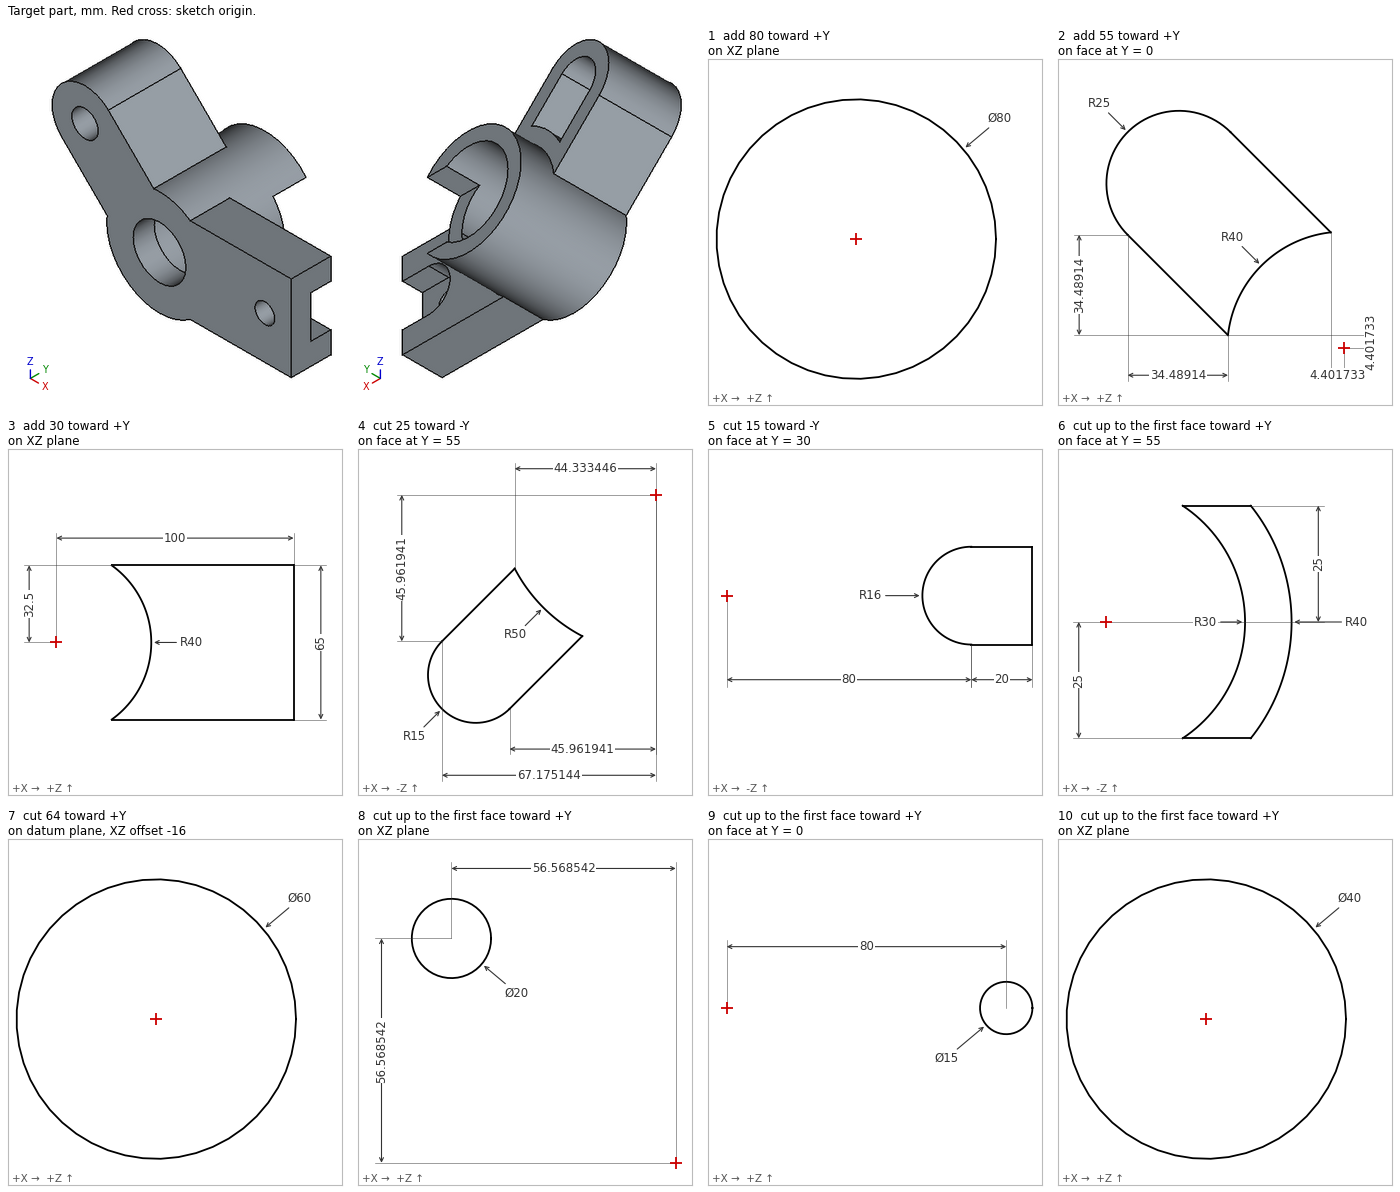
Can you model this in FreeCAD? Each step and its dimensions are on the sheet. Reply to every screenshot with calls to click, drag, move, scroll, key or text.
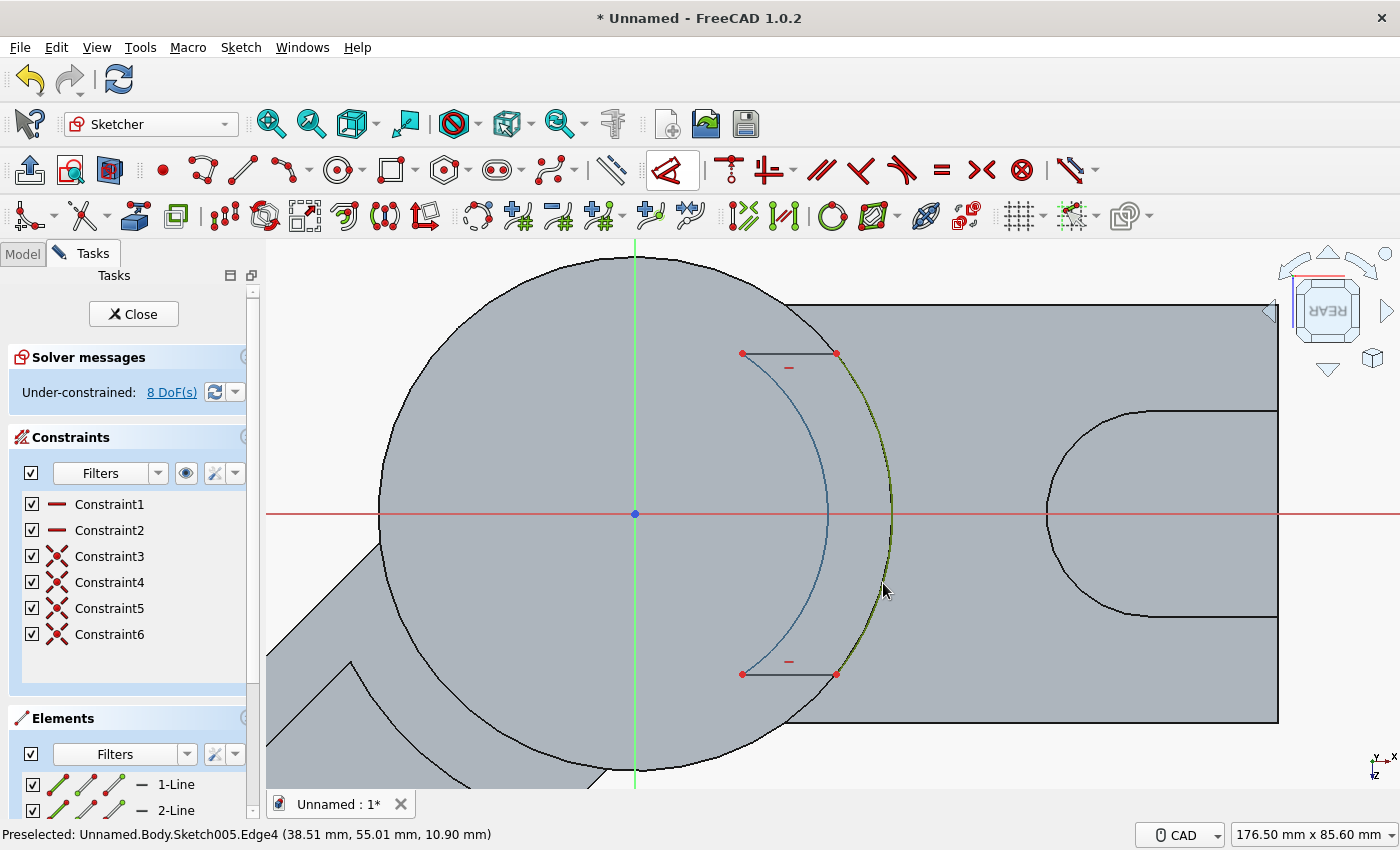
click(730, 170)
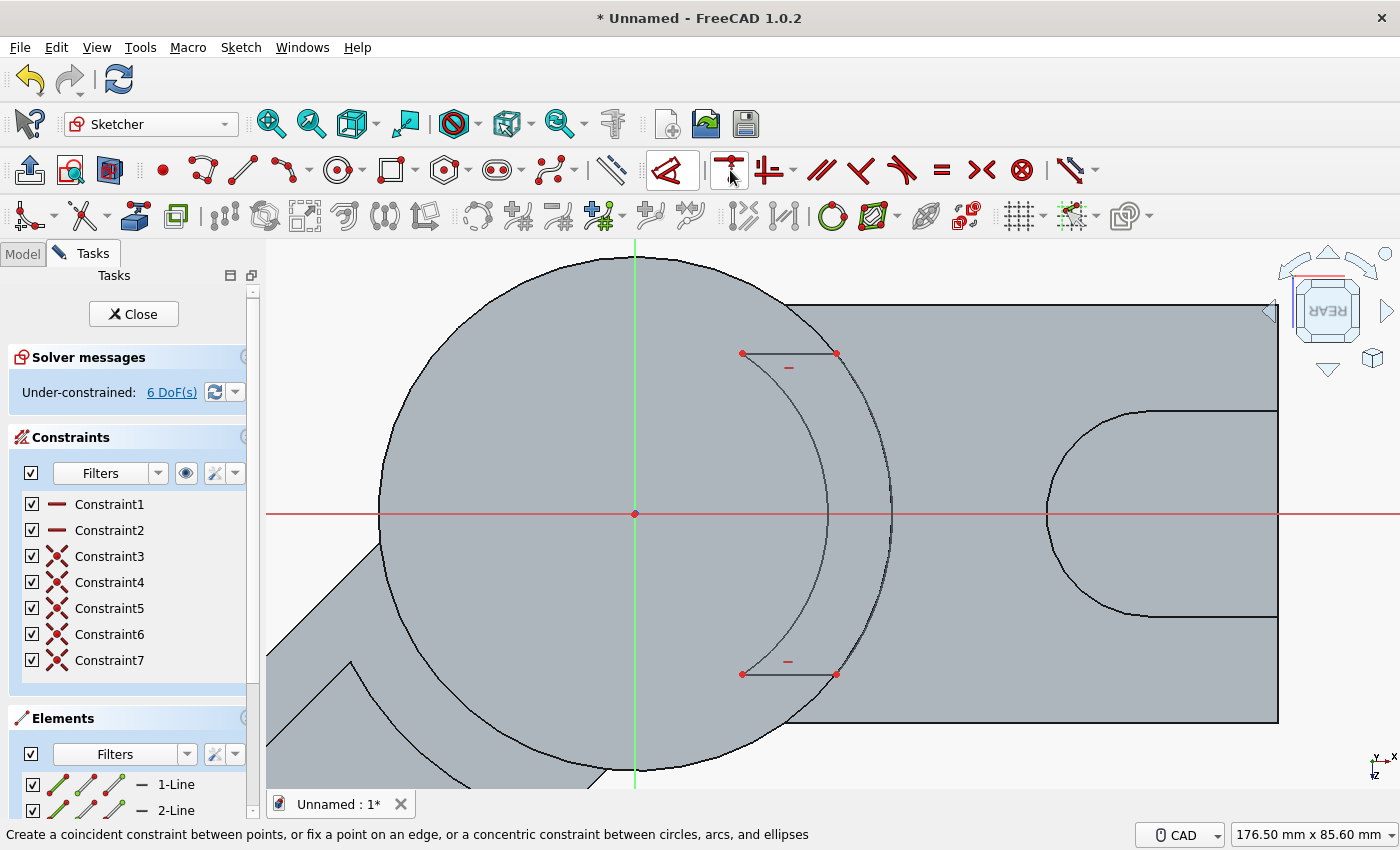
drag(625, 504, 645, 524)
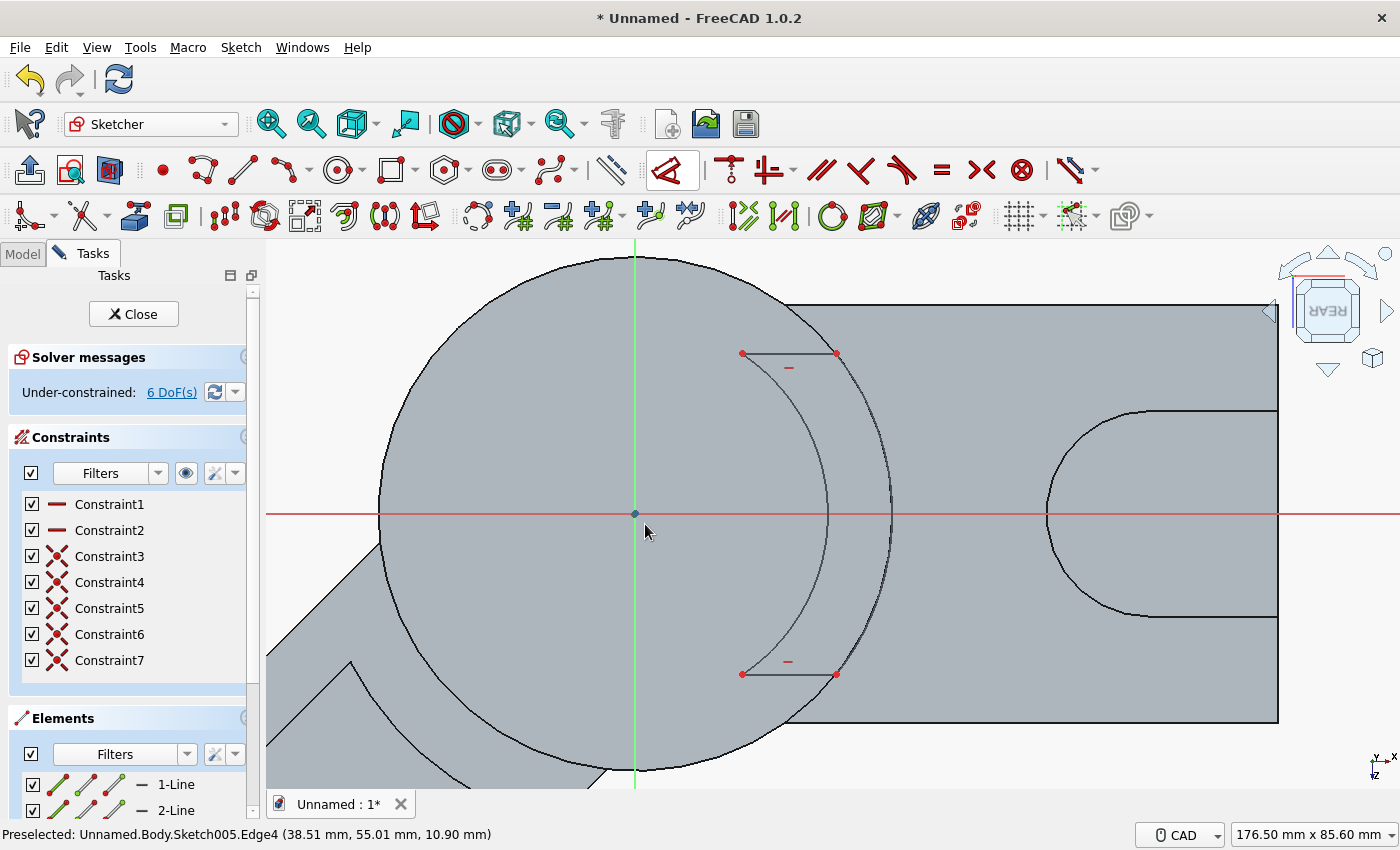
click(730, 170)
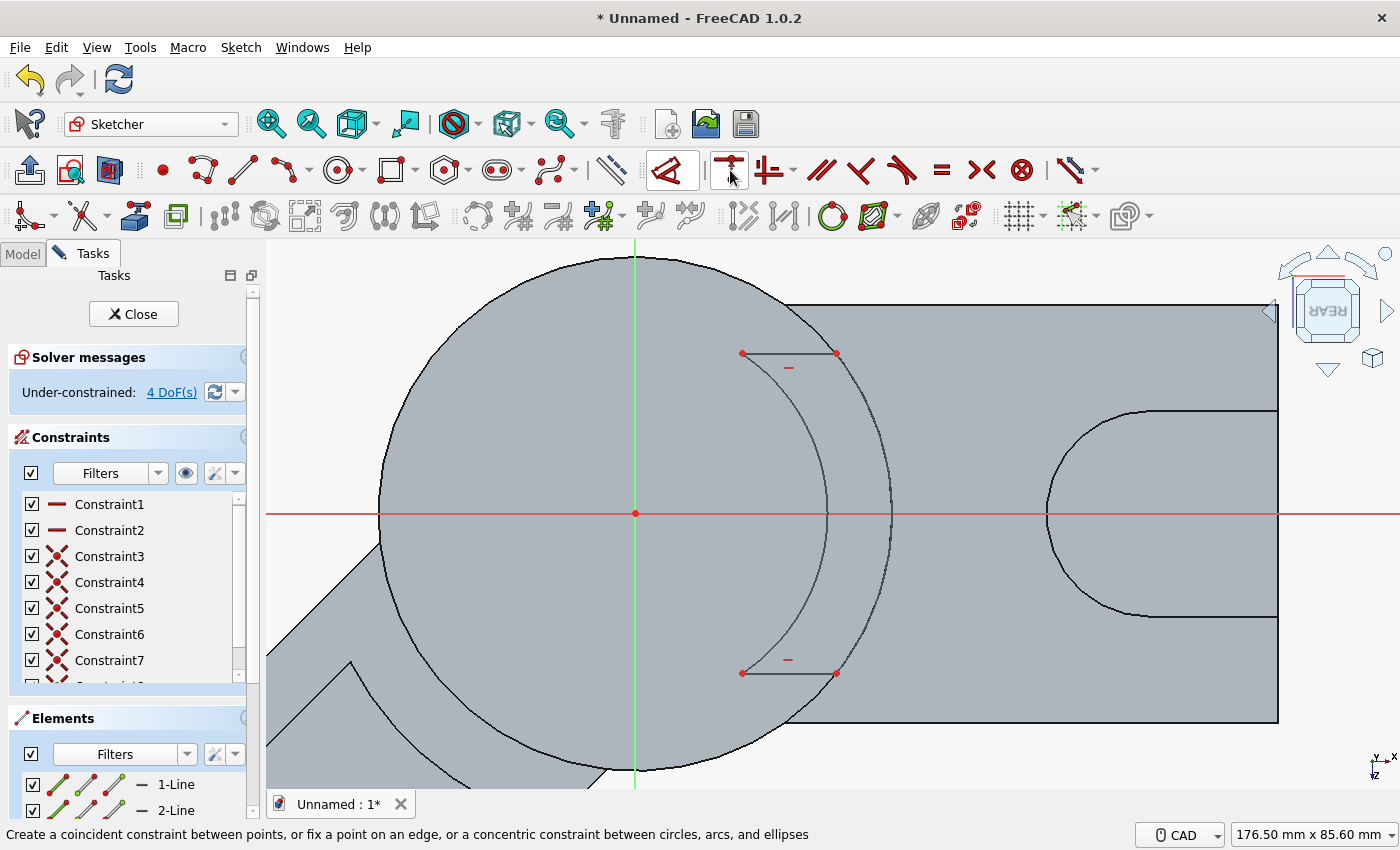
click(813, 587)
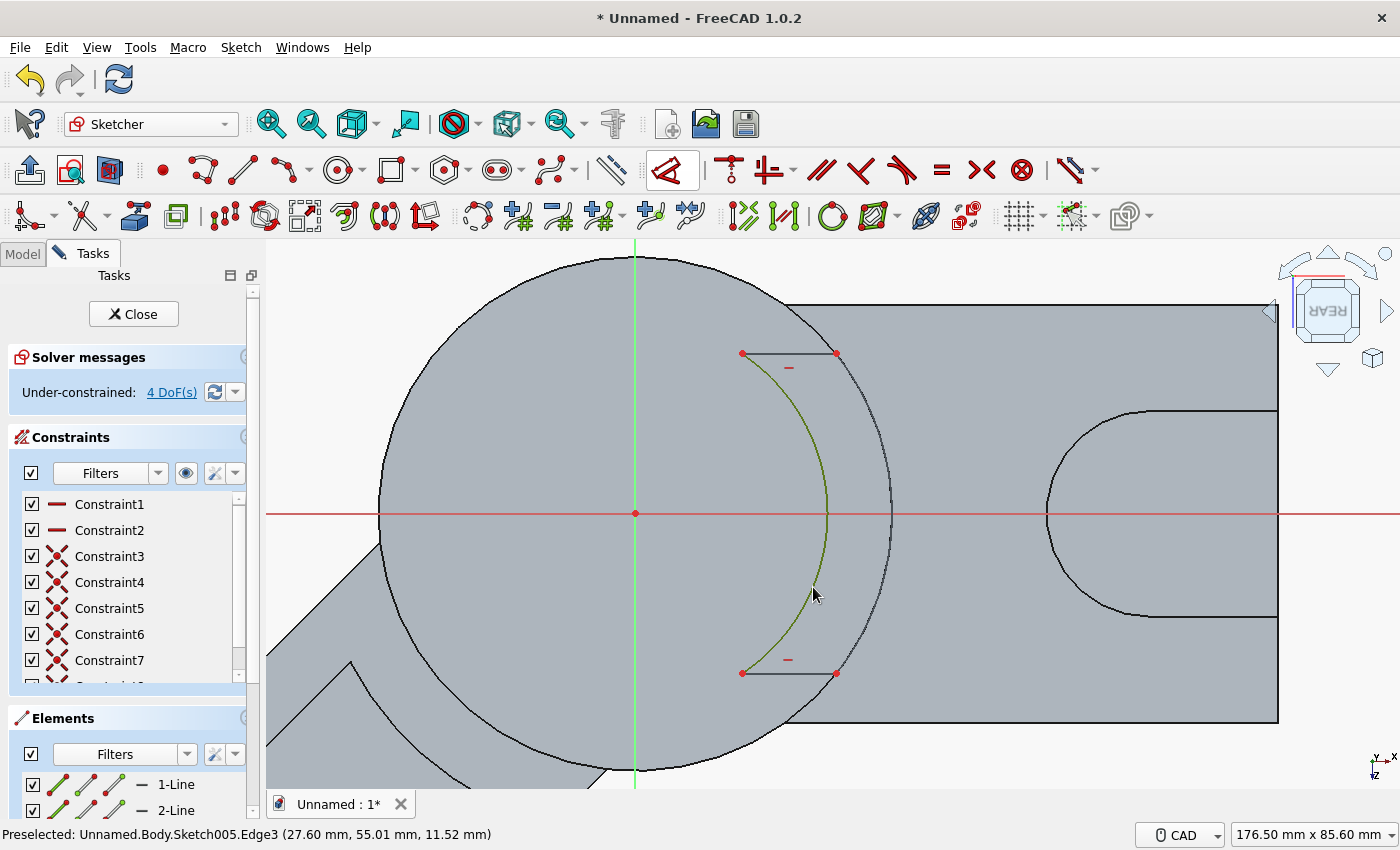
key(k)
key(r)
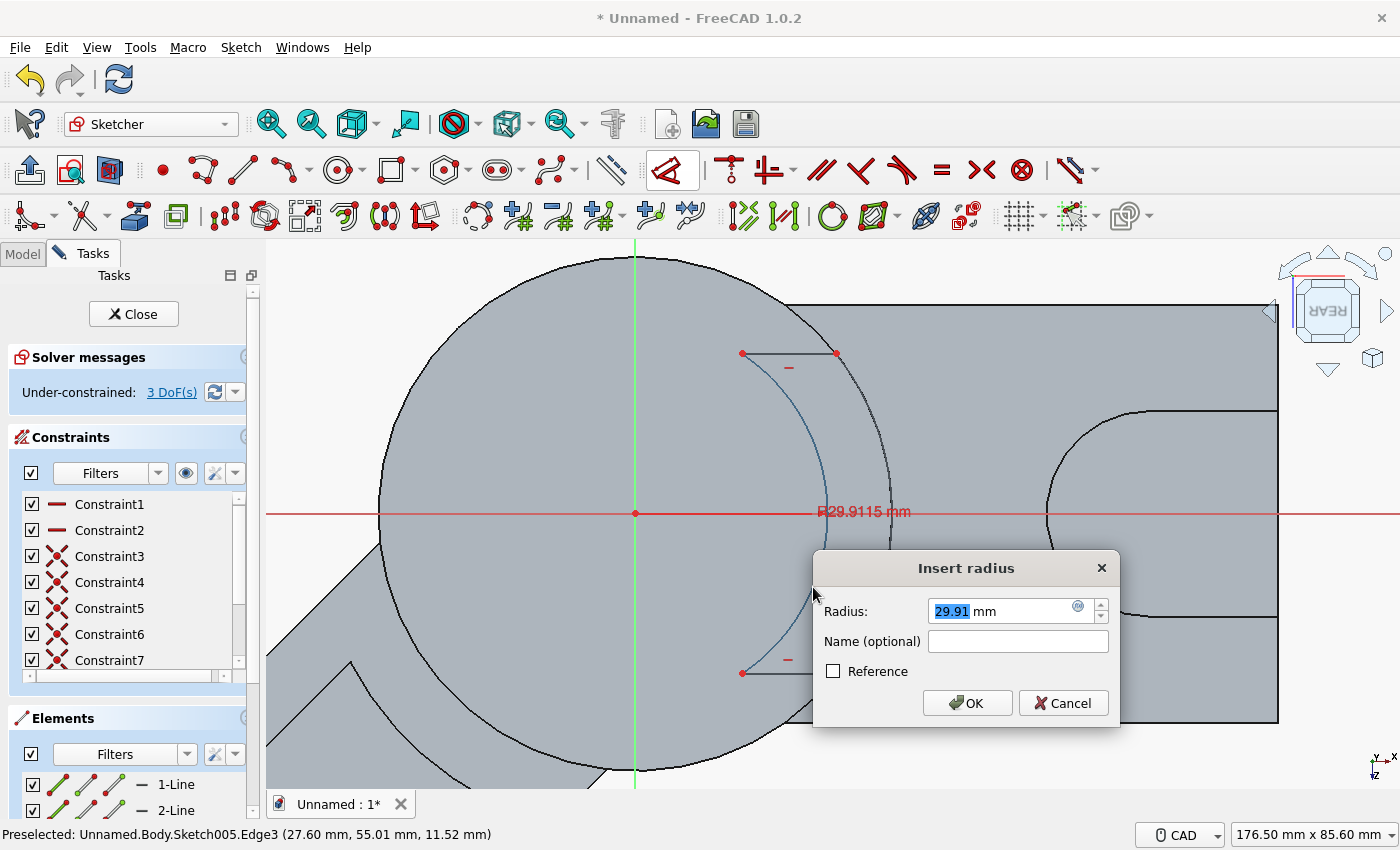
text(30)
key(Return)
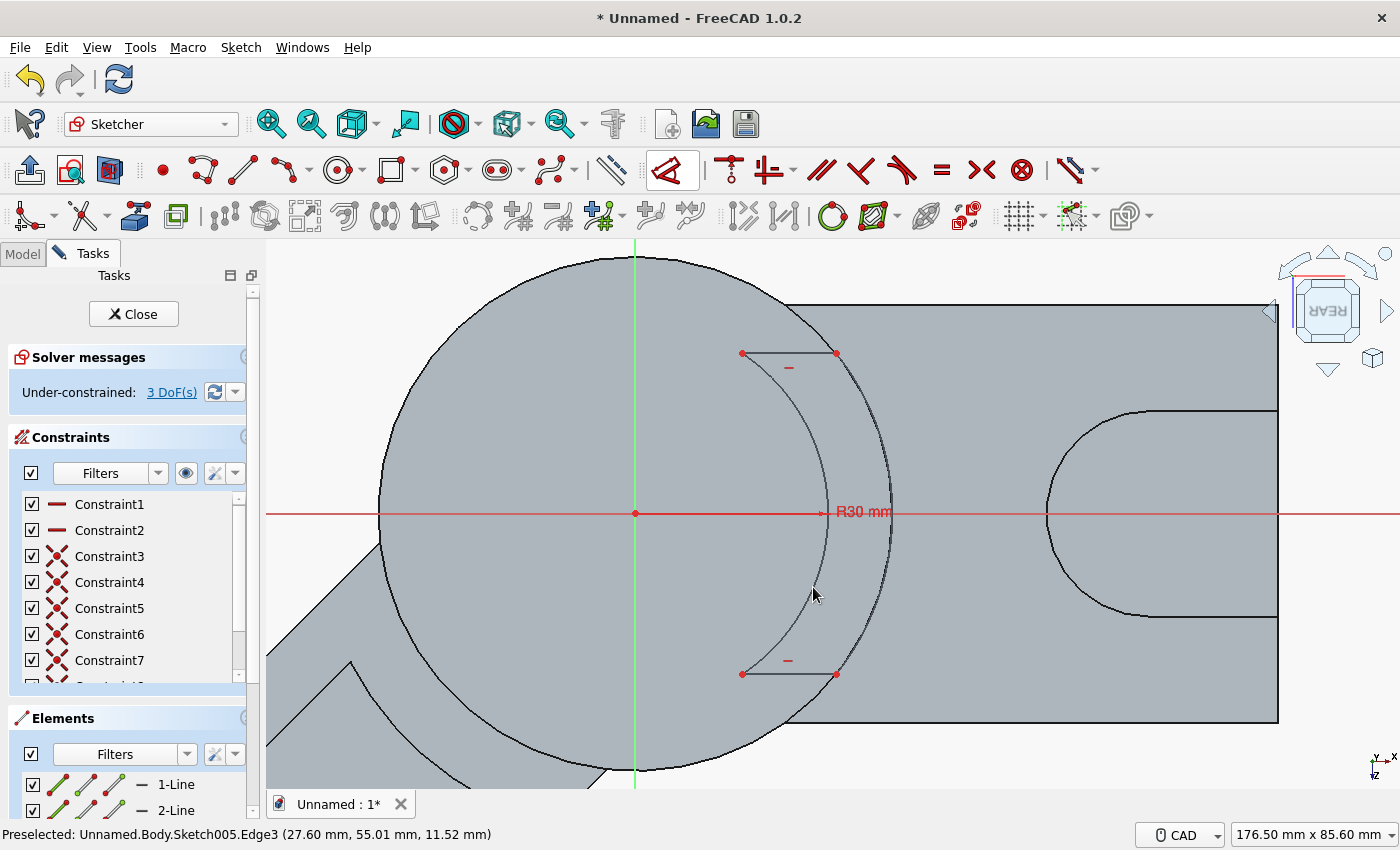
click(883, 582)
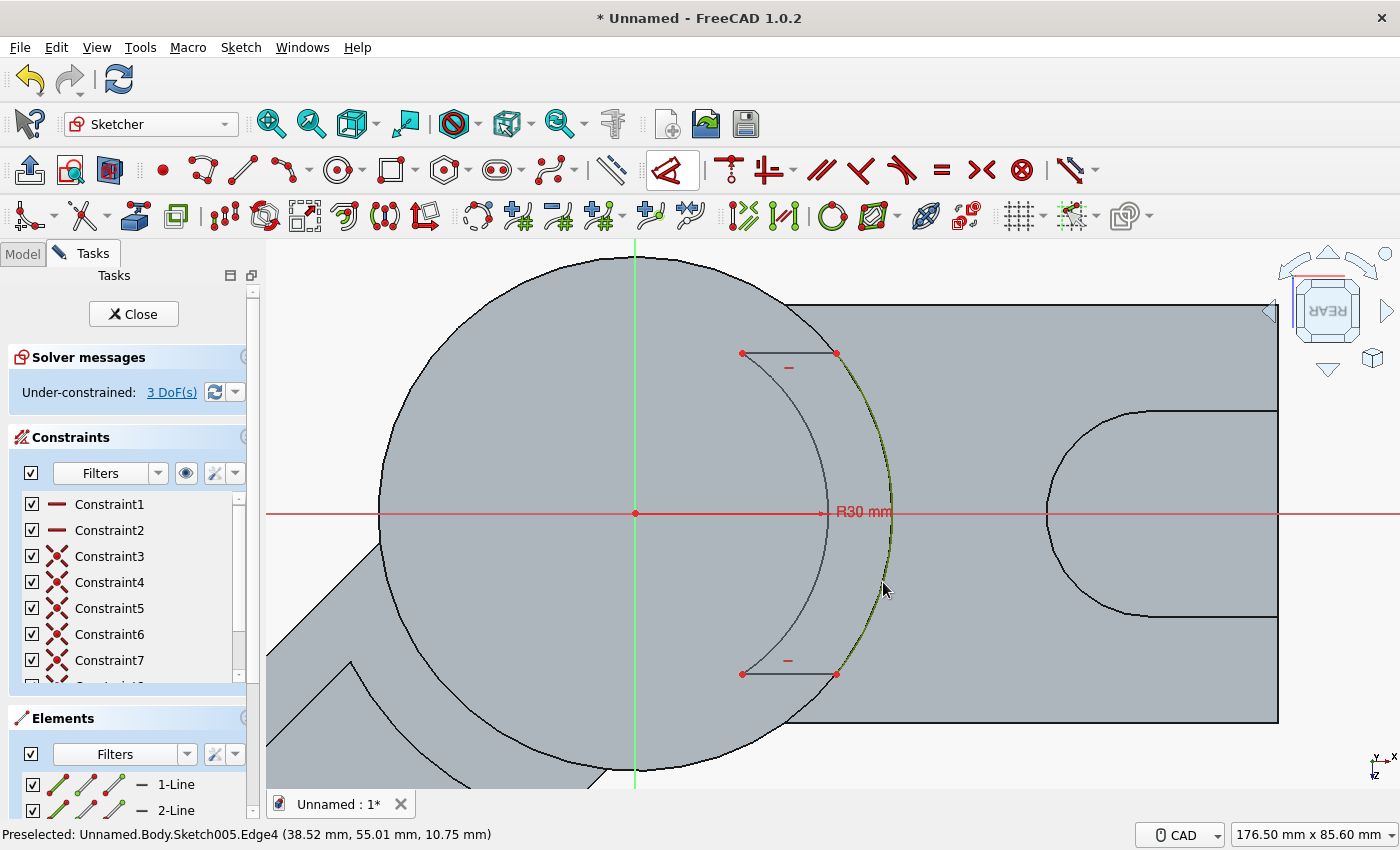
key(k)
key(r)